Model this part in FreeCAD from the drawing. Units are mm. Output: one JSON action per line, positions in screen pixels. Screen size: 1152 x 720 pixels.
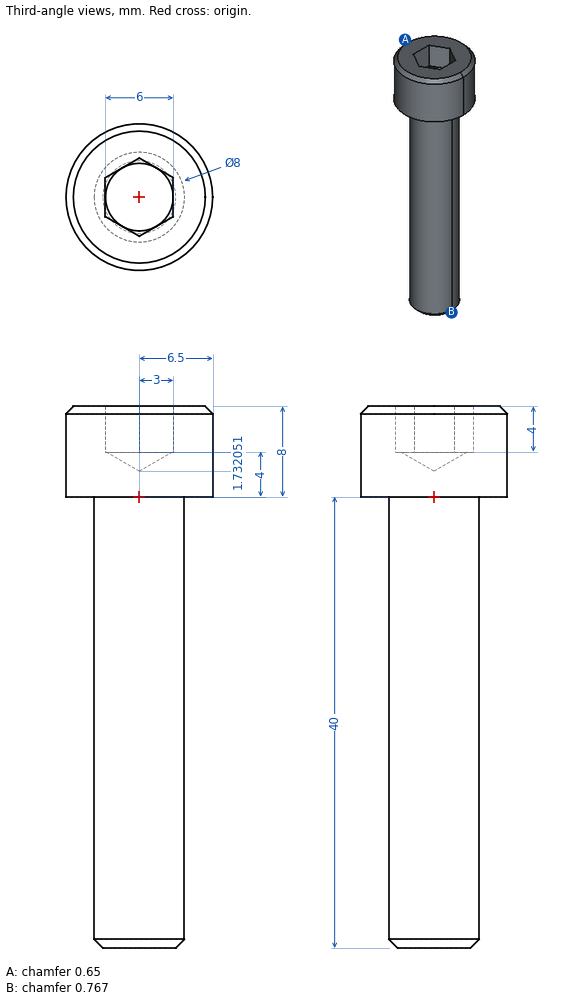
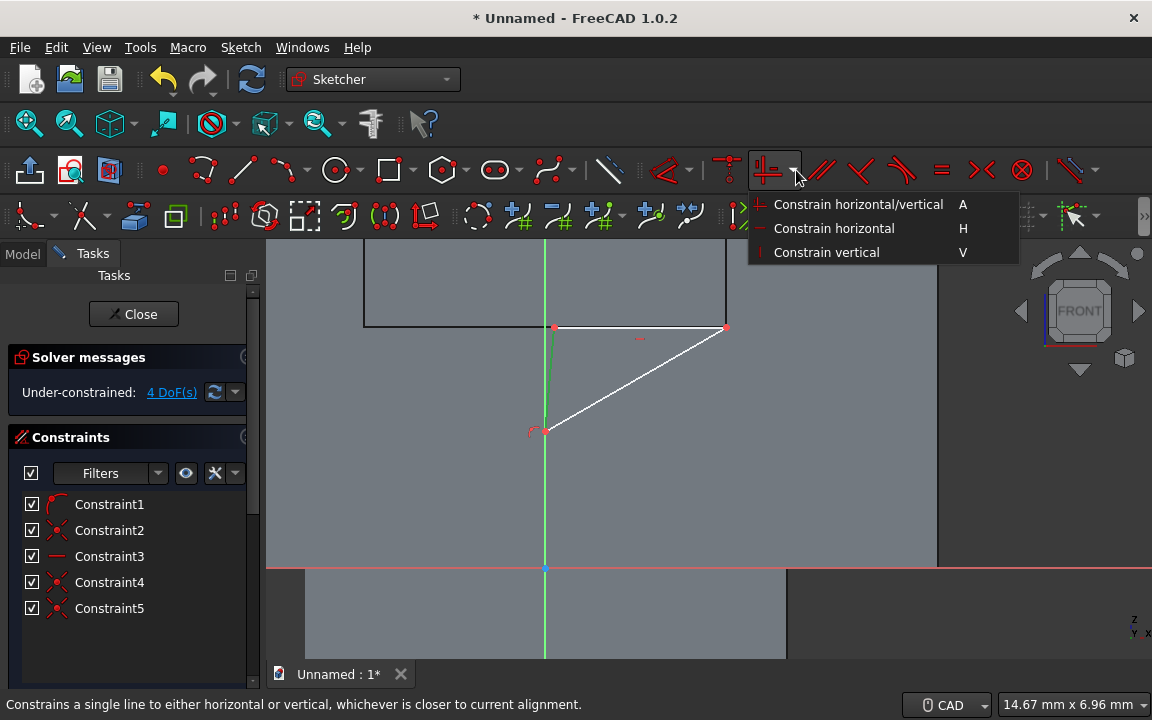
{"action": "left_click", "coordinate": [884, 252]}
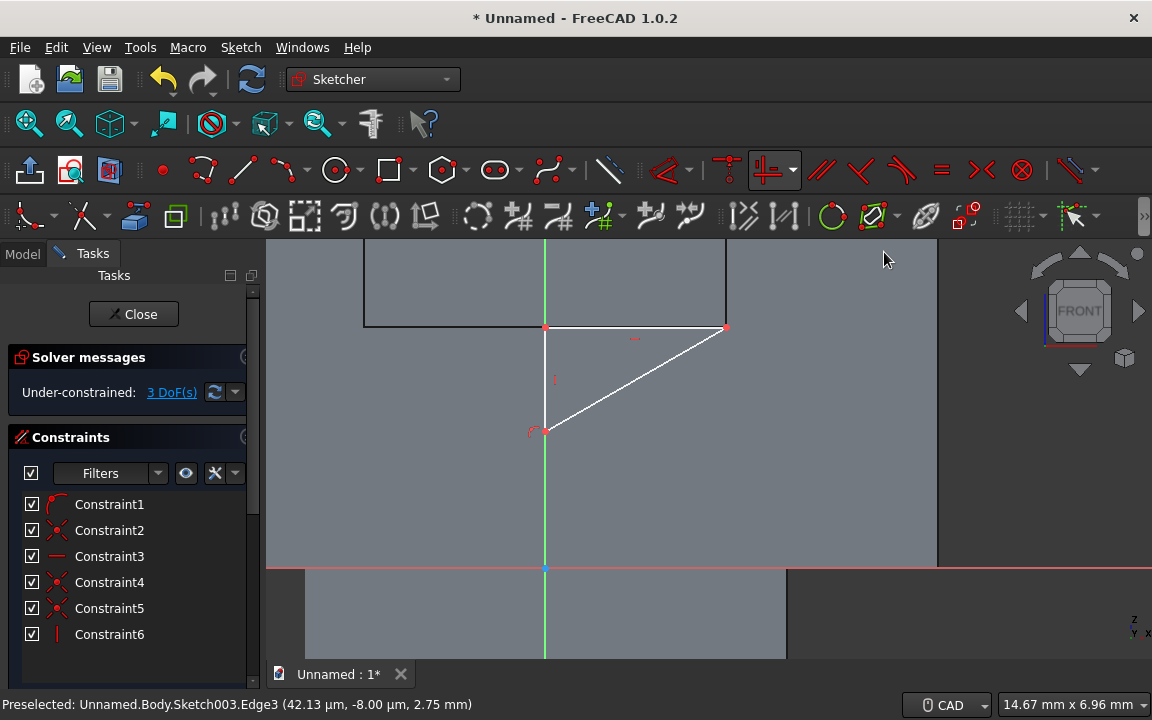
{"action": "left_click", "coordinate": [664, 170]}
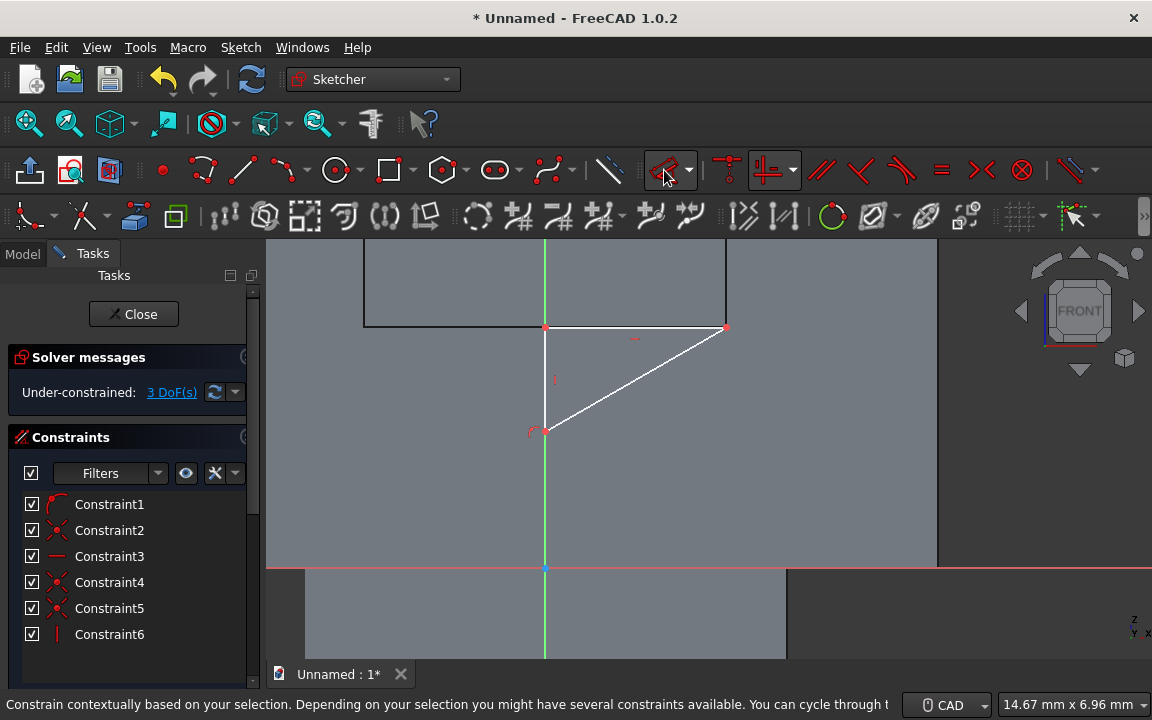
{"action": "left_click", "coordinate": [672, 328]}
{"action": "left_click", "coordinate": [636, 294]}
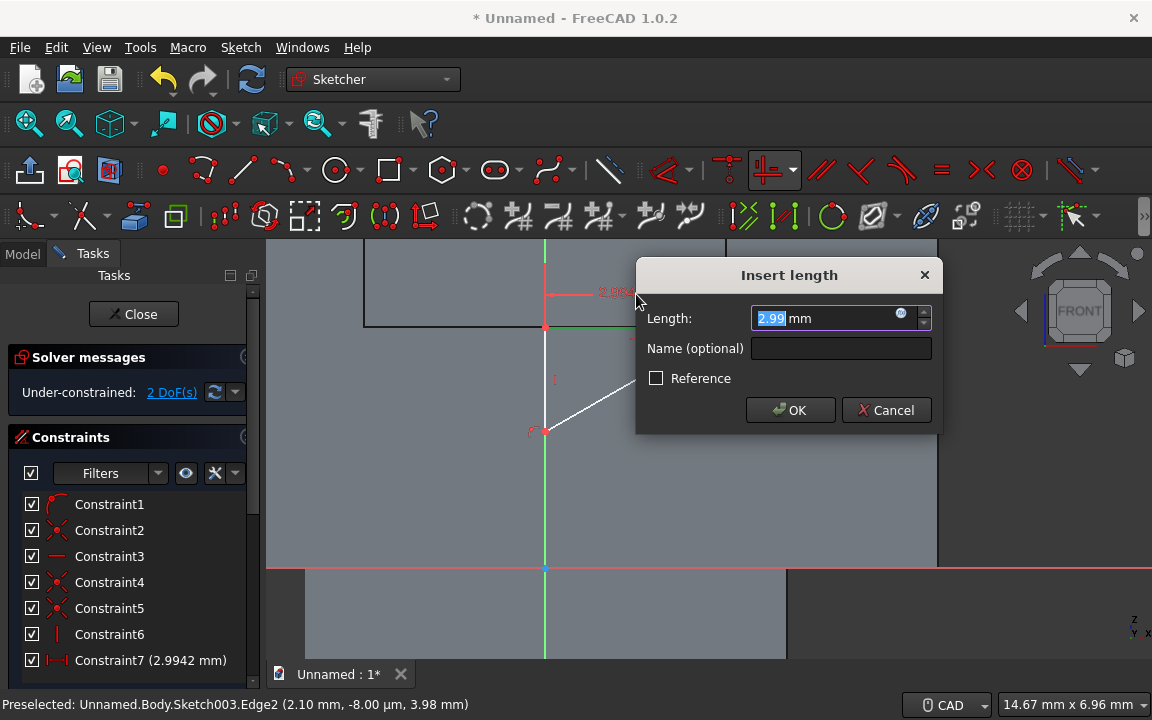
{"action": "type", "text": "3"}
{"action": "key", "text": "Return"}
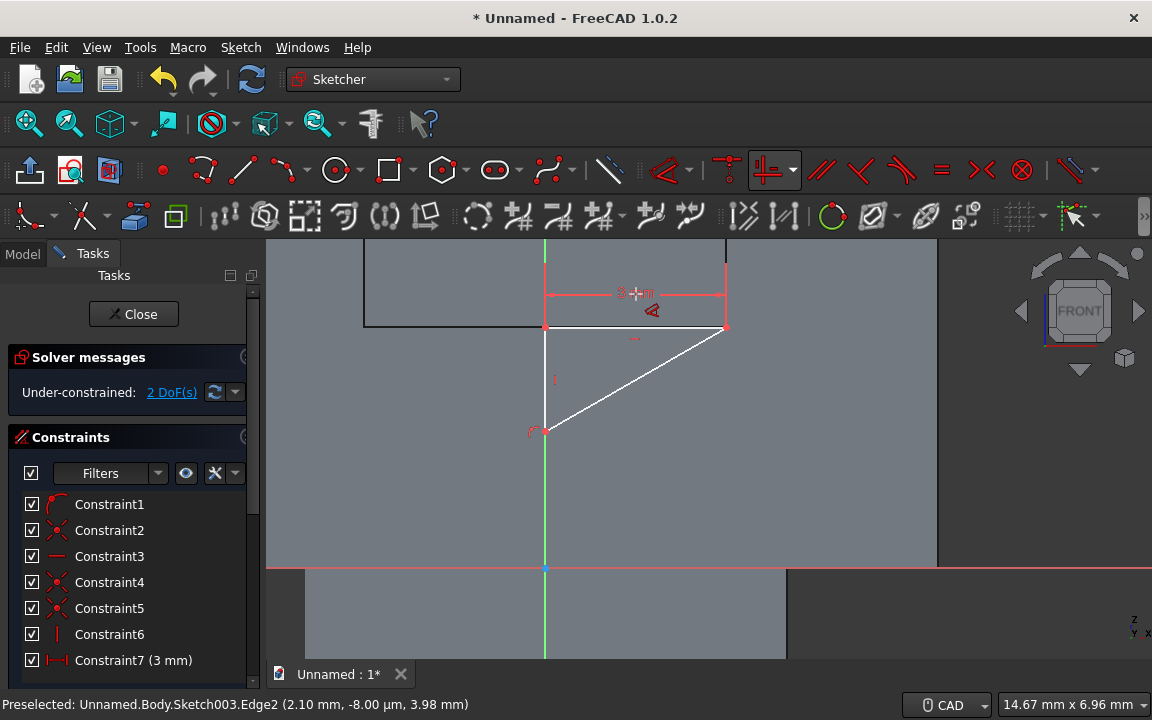
{"action": "left_click", "coordinate": [726, 328]}
{"action": "left_click", "coordinate": [760, 448]}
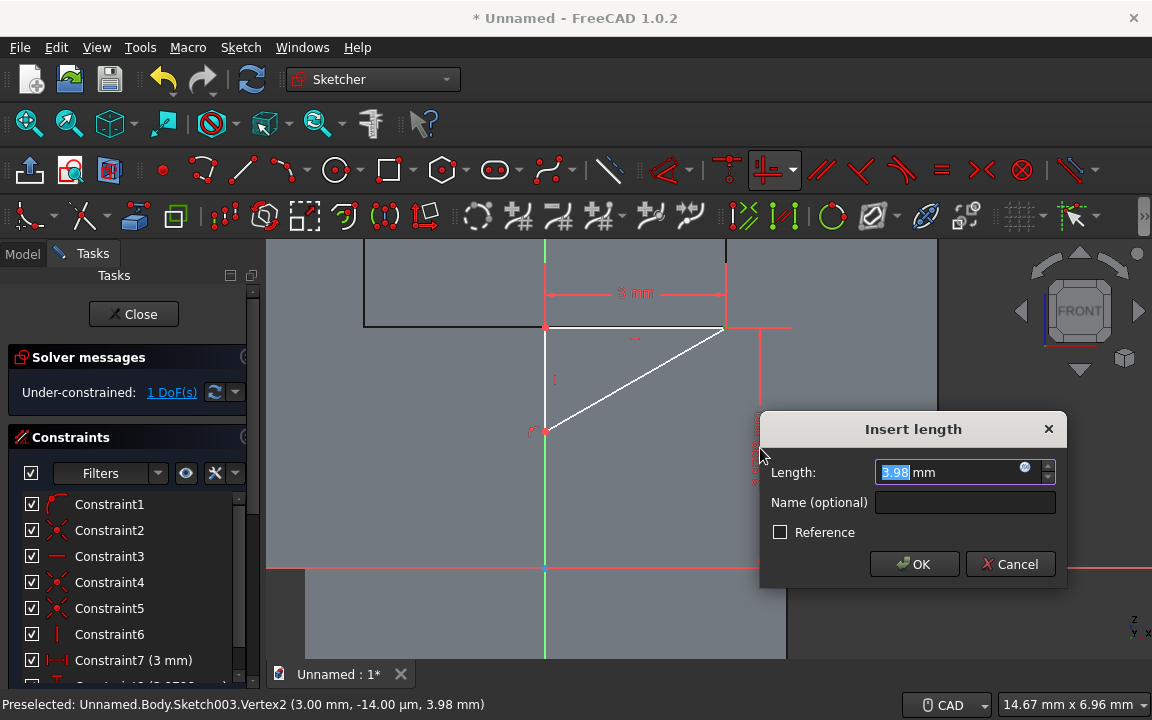
{"action": "type", "text": "4"}
{"action": "key", "text": "Return"}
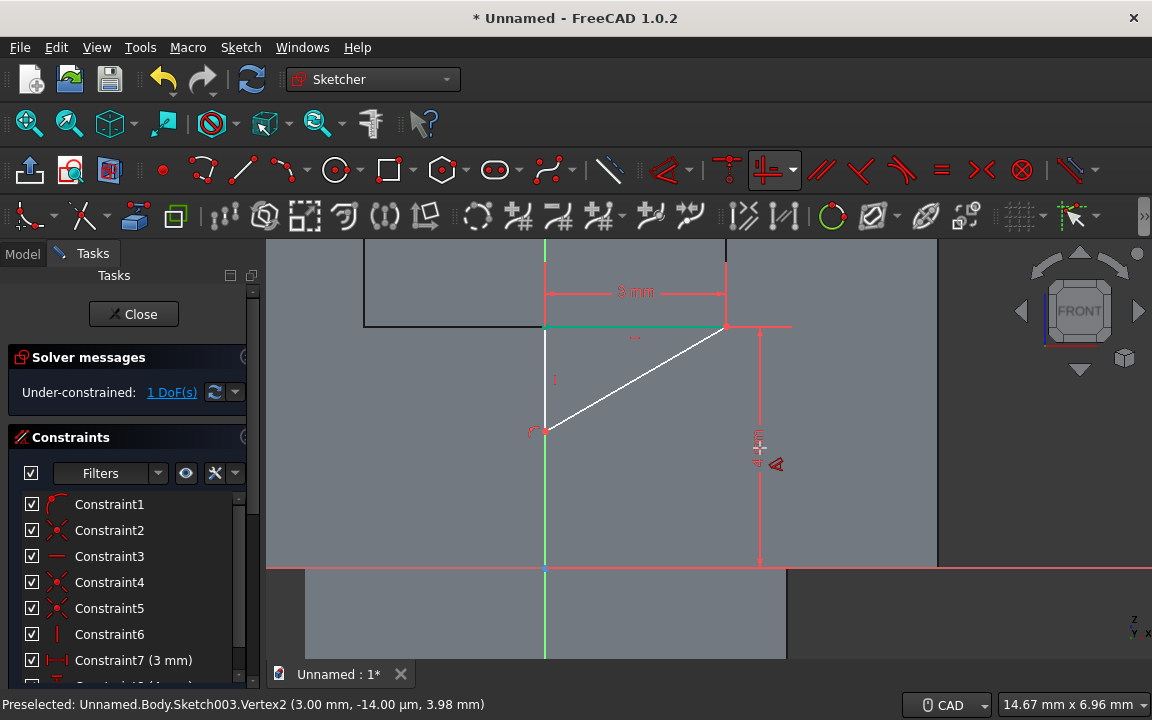
{"action": "left_click", "coordinate": [545, 358]}
{"action": "left_click", "coordinate": [511, 379]}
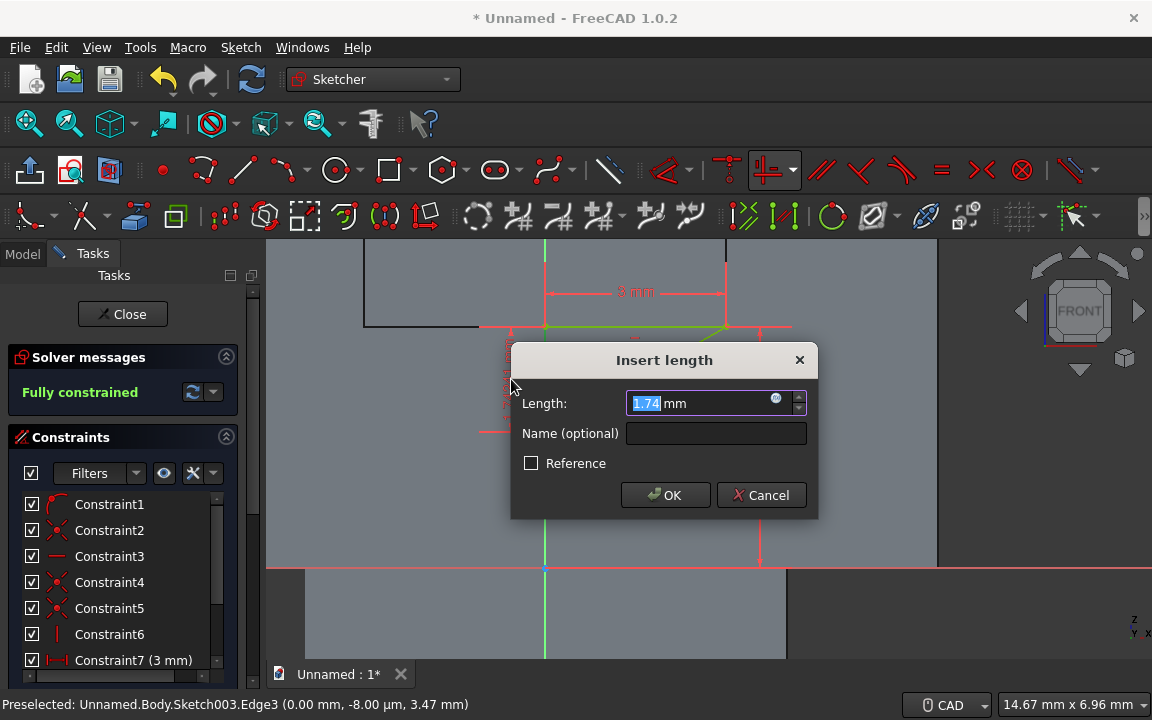
{"action": "type", "text": "1.732051"}
{"action": "key", "text": "Return"}
{"action": "key", "text": "Escape"}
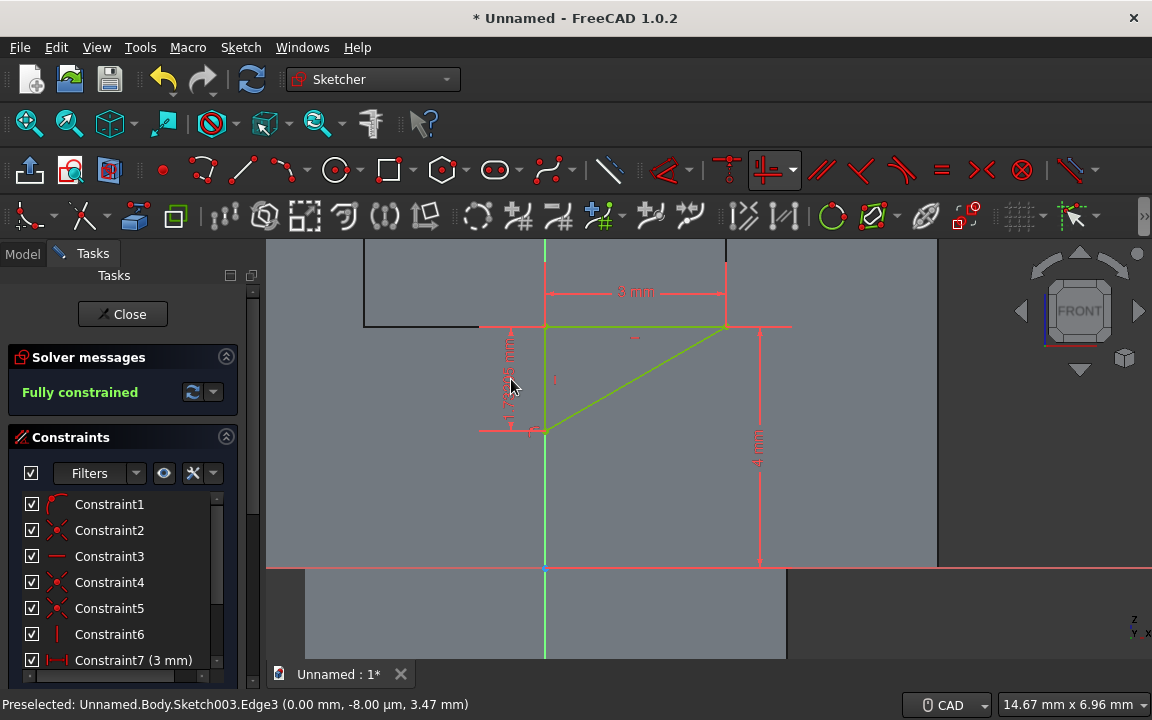
{"action": "left_click", "coordinate": [123, 314]}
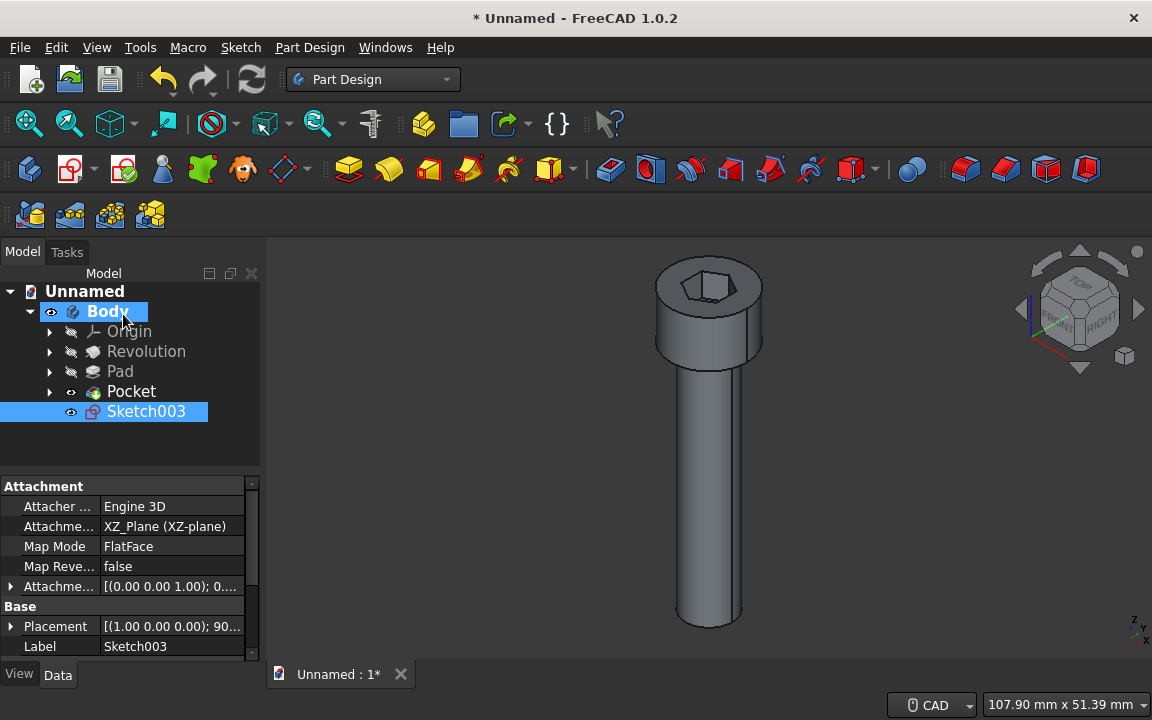
{"action": "left_click", "coordinate": [692, 170]}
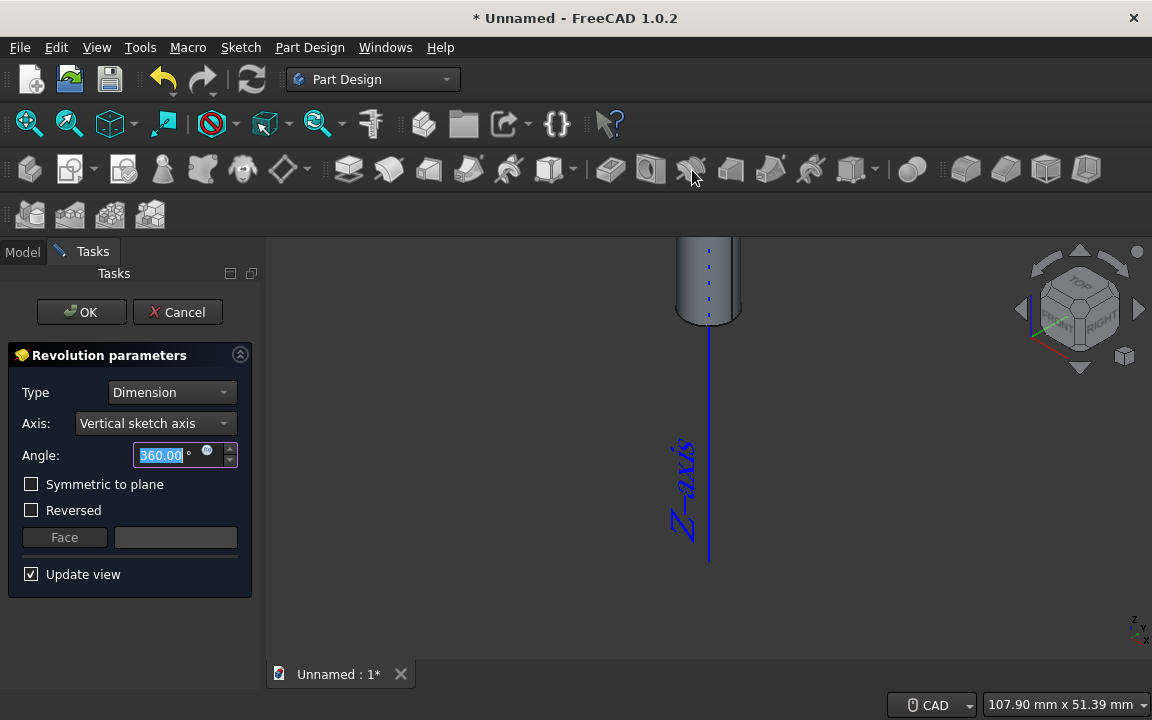
{"action": "left_click", "coordinate": [82, 312]}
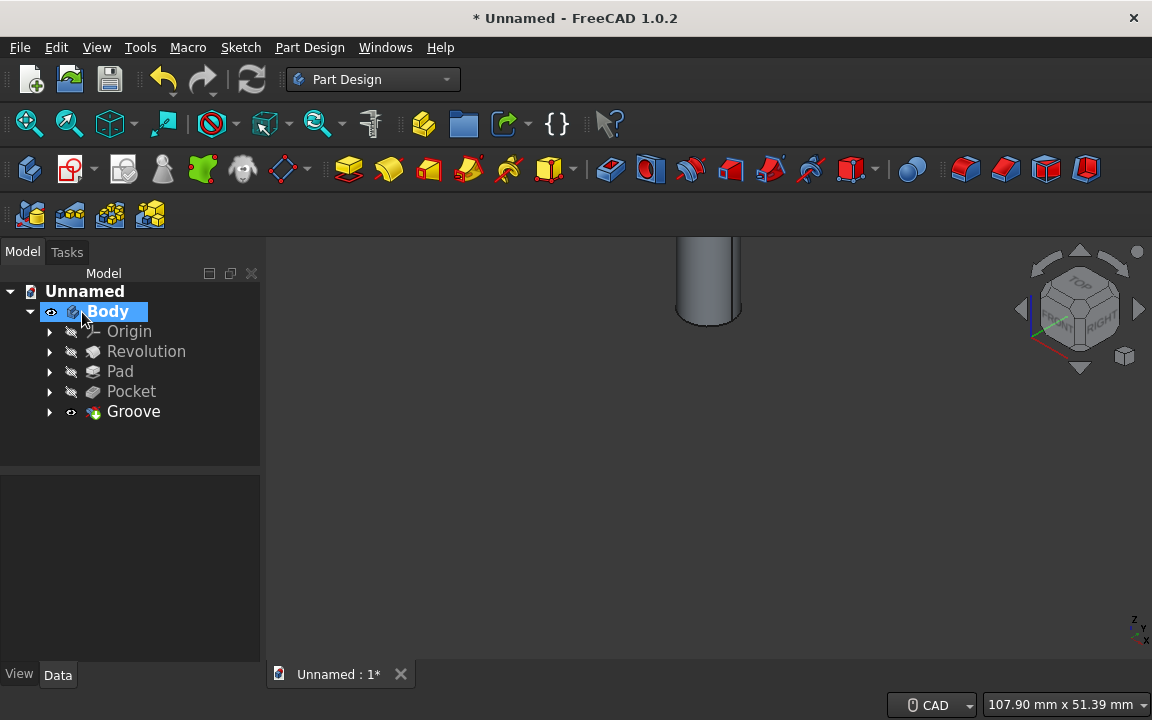
{"action": "left_click", "coordinate": [30, 124]}